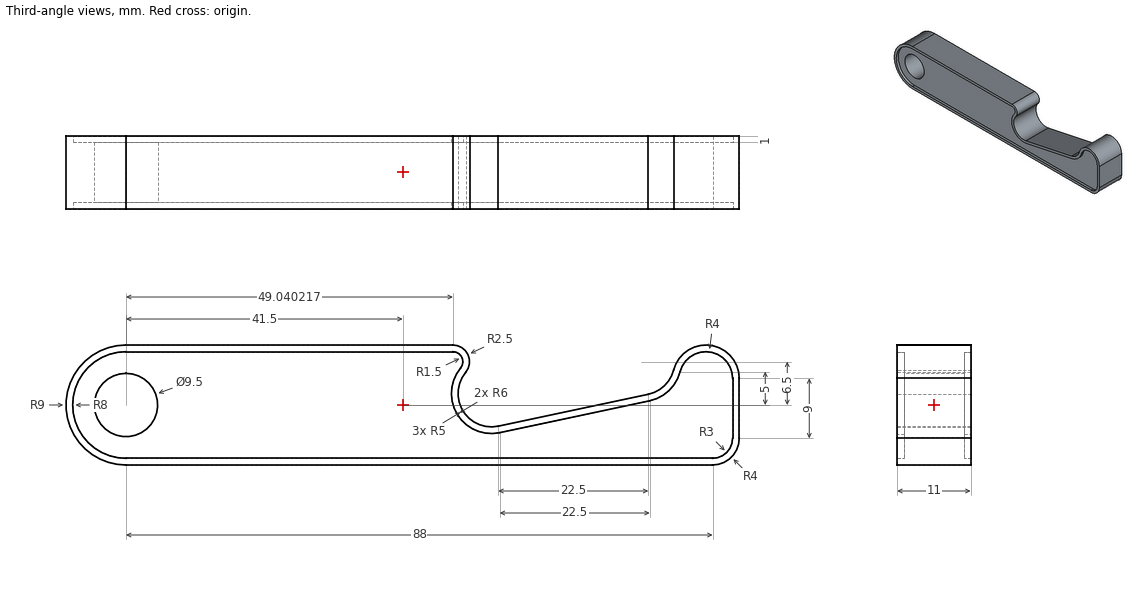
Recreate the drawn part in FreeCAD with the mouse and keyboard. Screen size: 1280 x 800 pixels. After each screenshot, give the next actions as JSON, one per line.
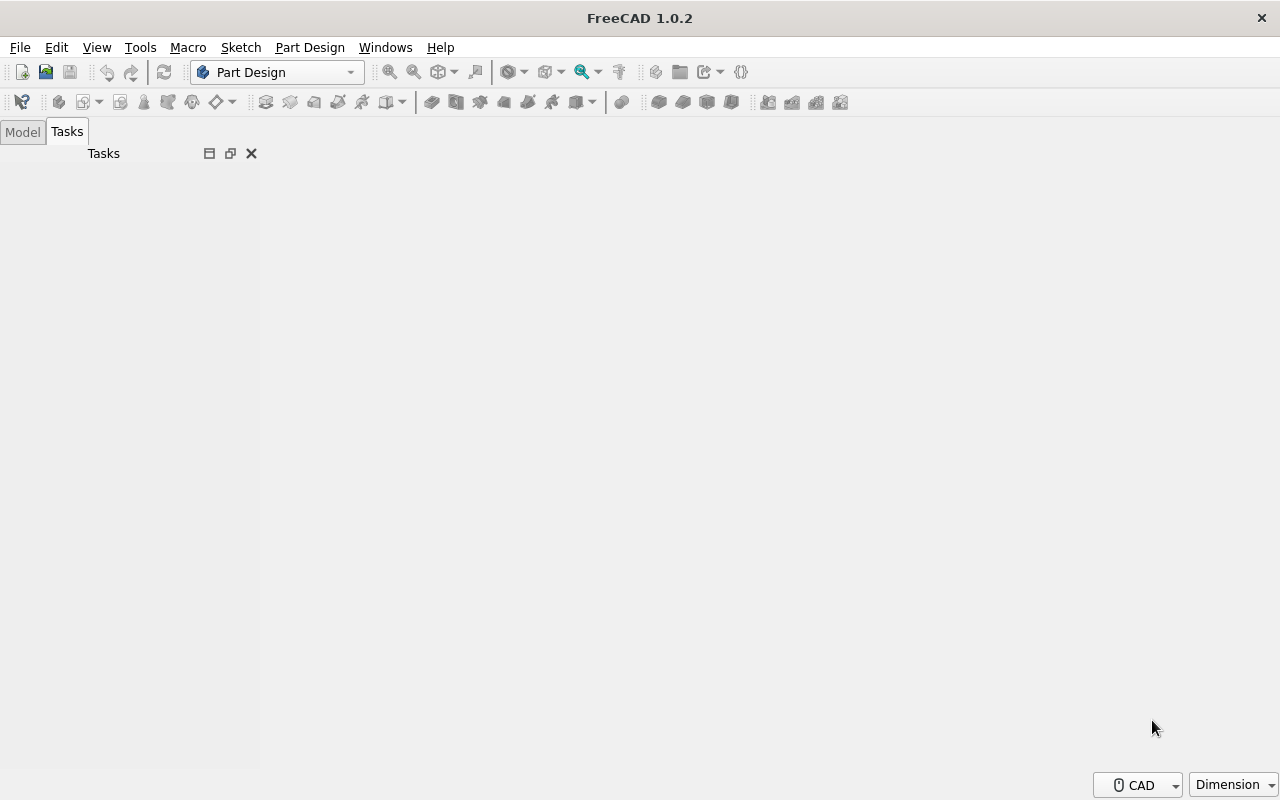
{"action": "left_click", "coordinate": [700, 72]}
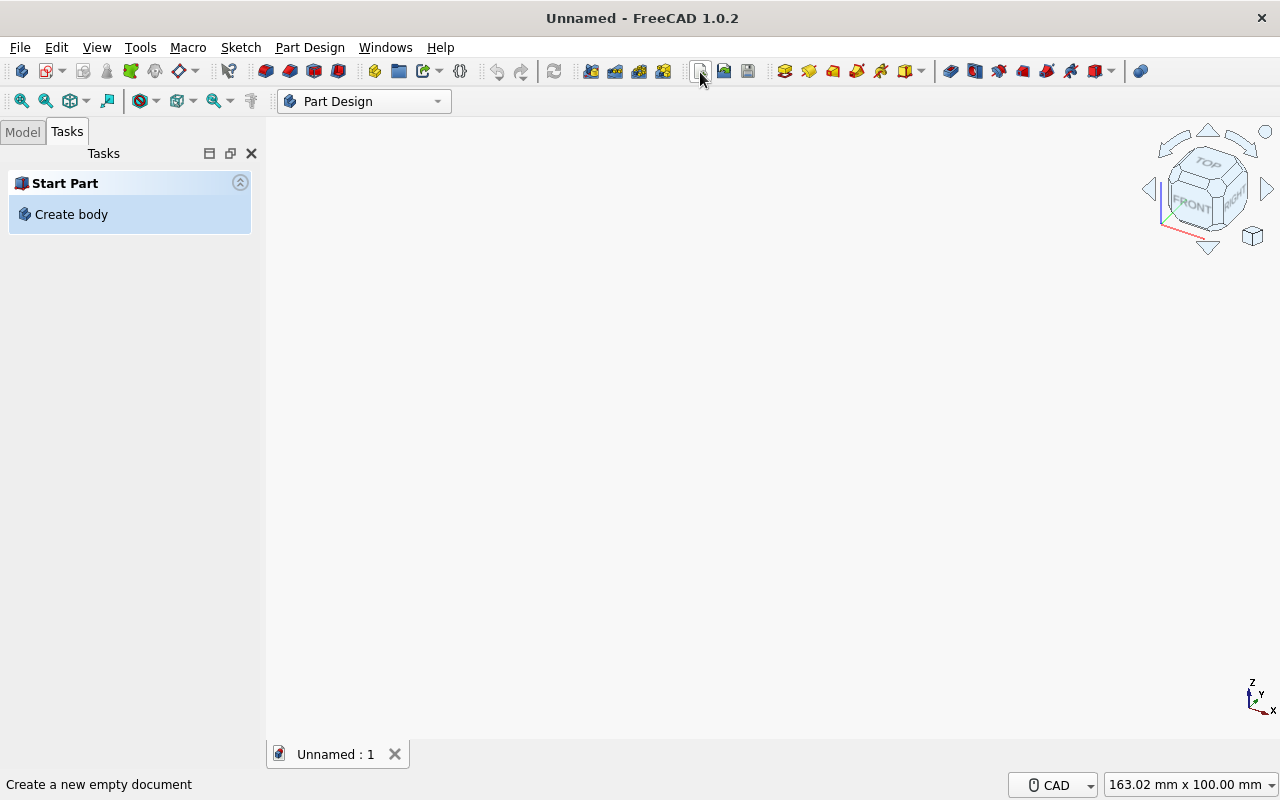
{"action": "left_click", "coordinate": [46, 72]}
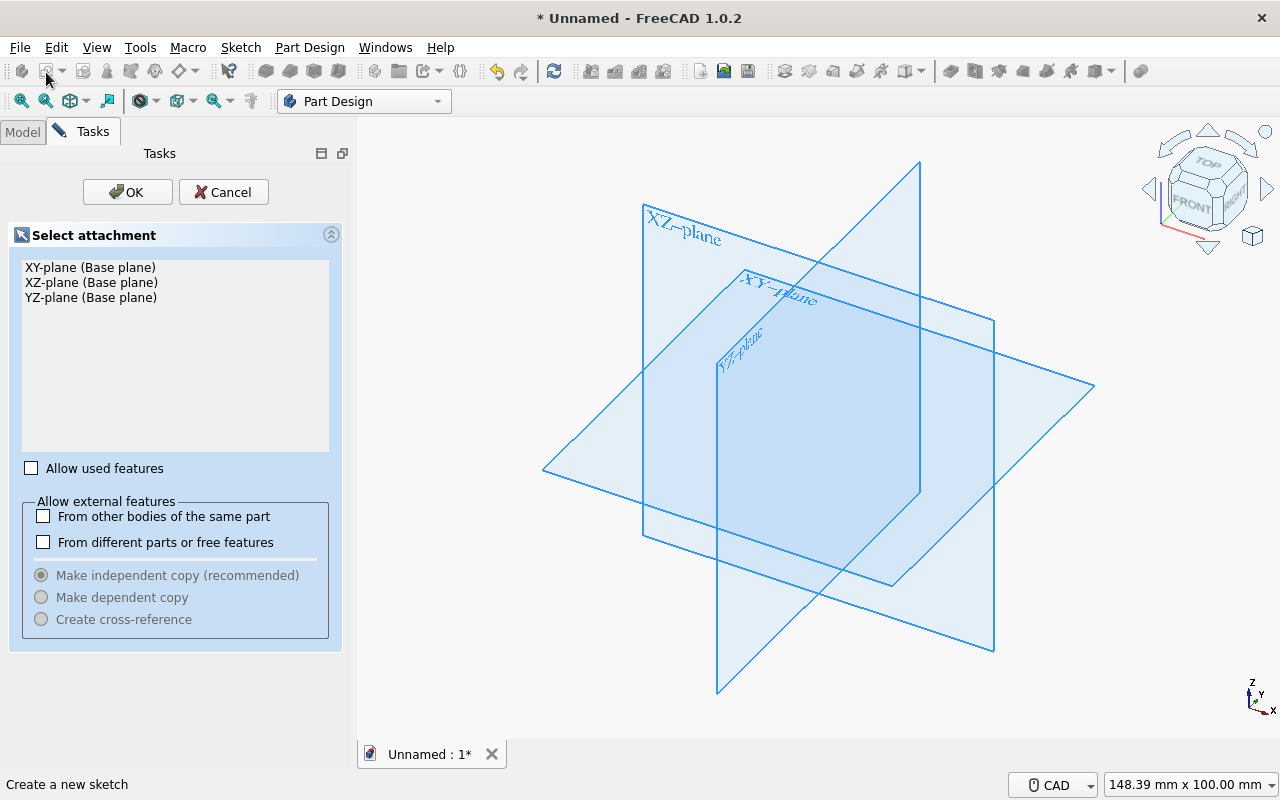
{"action": "left_click", "coordinate": [82, 282]}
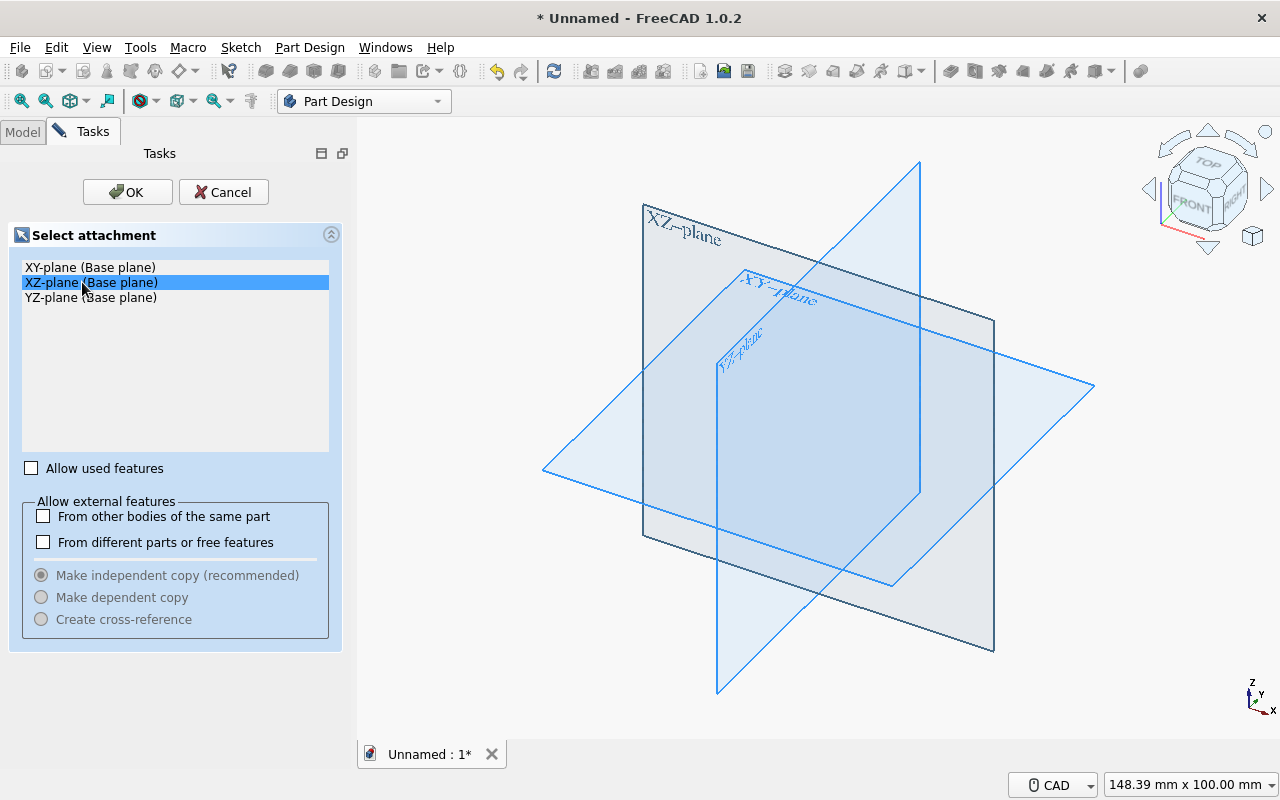
{"action": "left_click", "coordinate": [128, 192]}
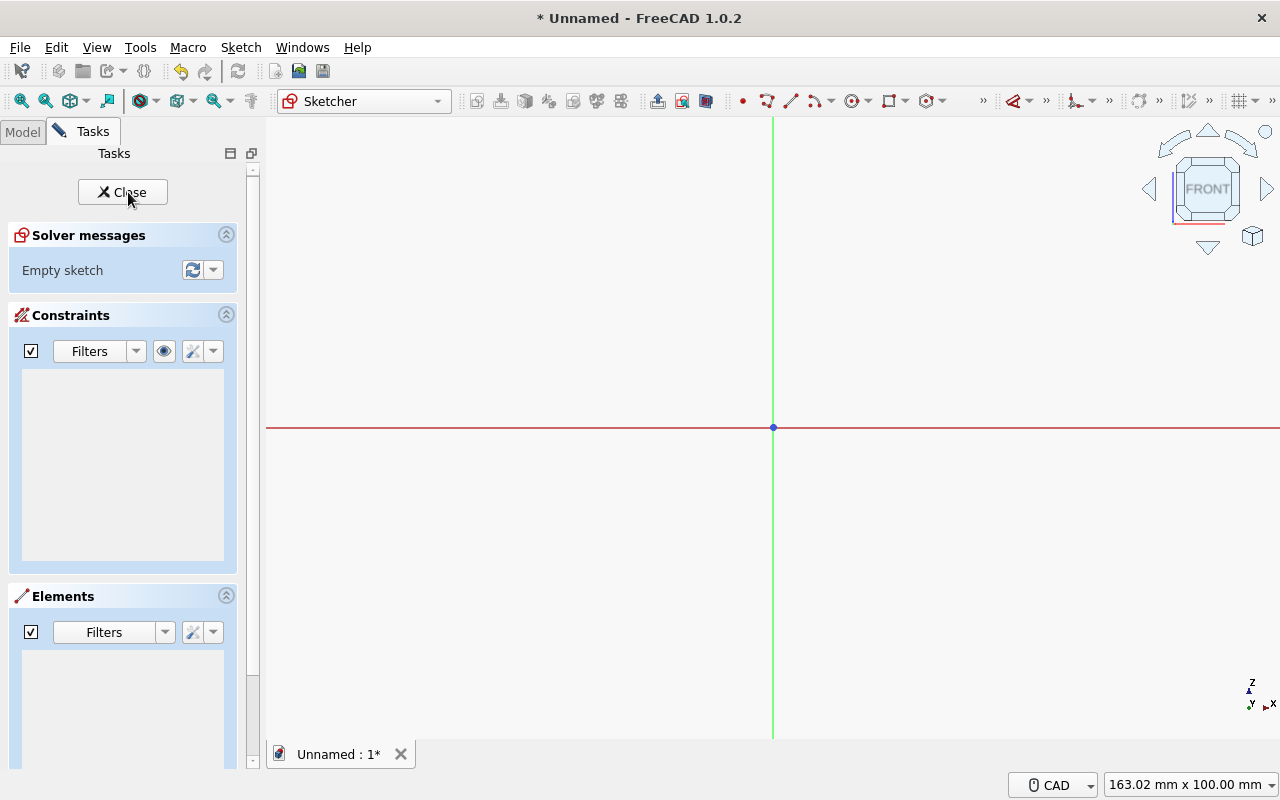
{"action": "left_click", "coordinate": [792, 102]}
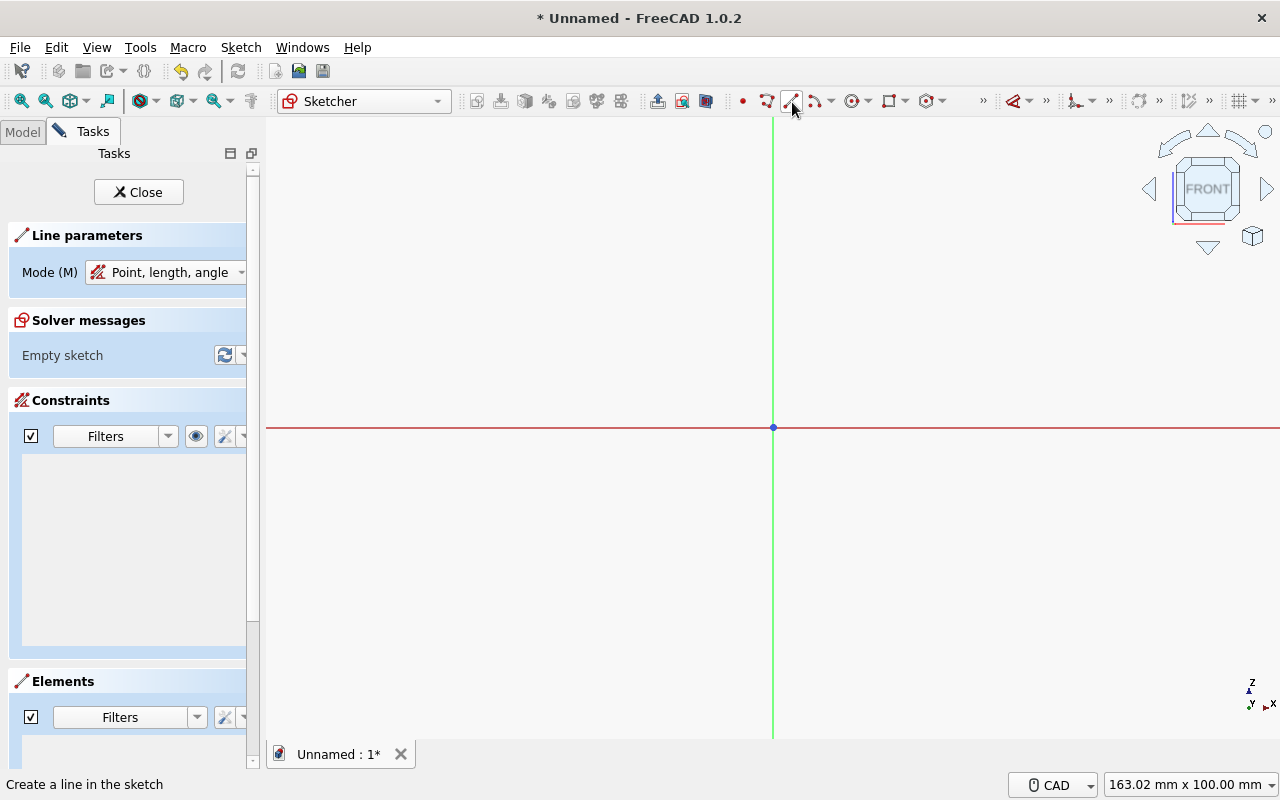
{"action": "left_click", "coordinate": [1062, 484]}
{"action": "left_click", "coordinate": [515, 484]}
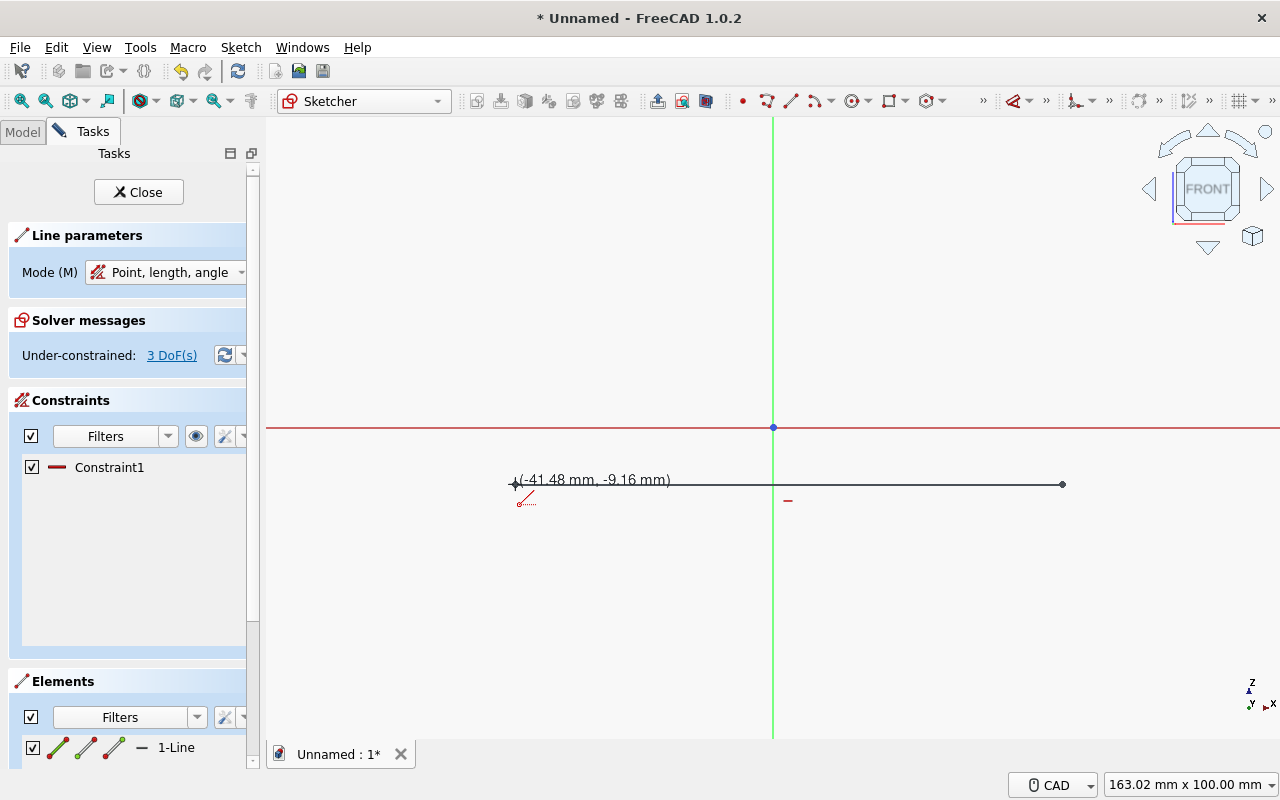
{"action": "left_click", "coordinate": [515, 372]}
{"action": "left_click", "coordinate": [820, 372]}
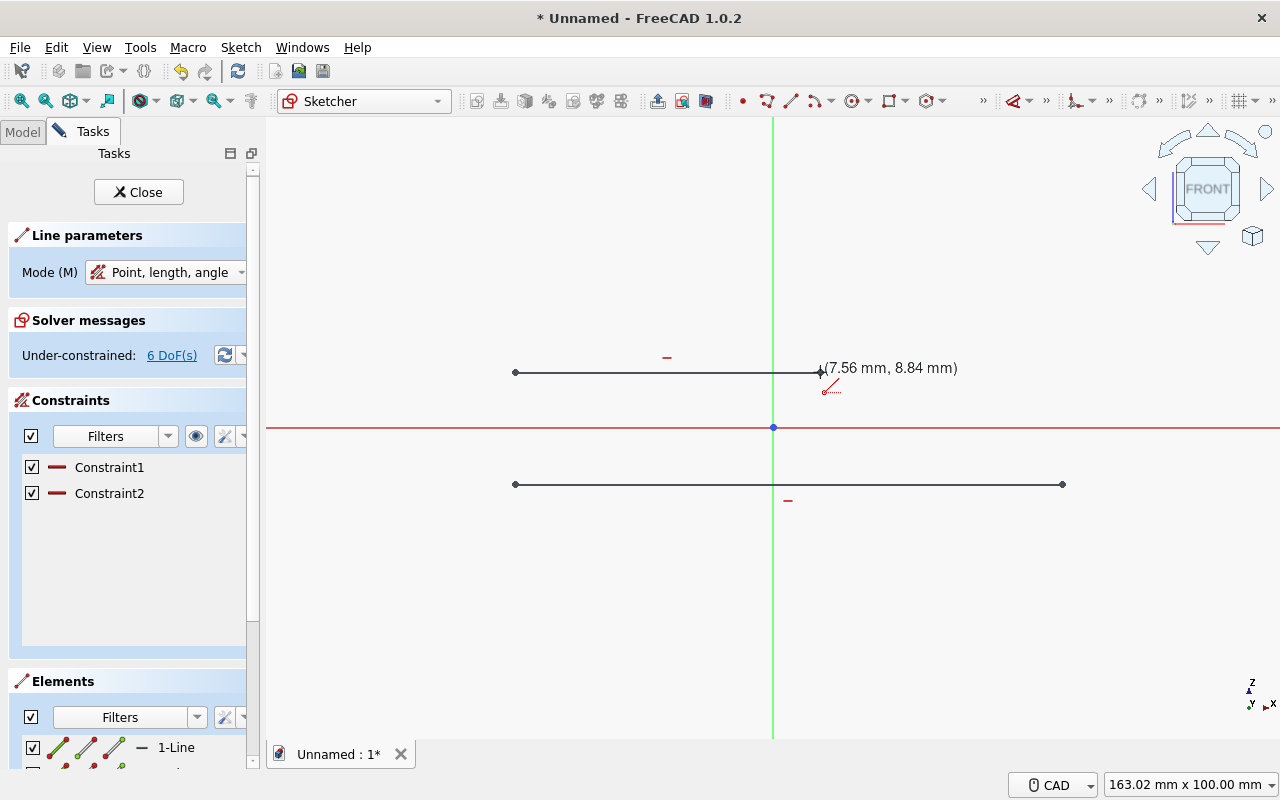
{"action": "left_click", "coordinate": [862, 448]}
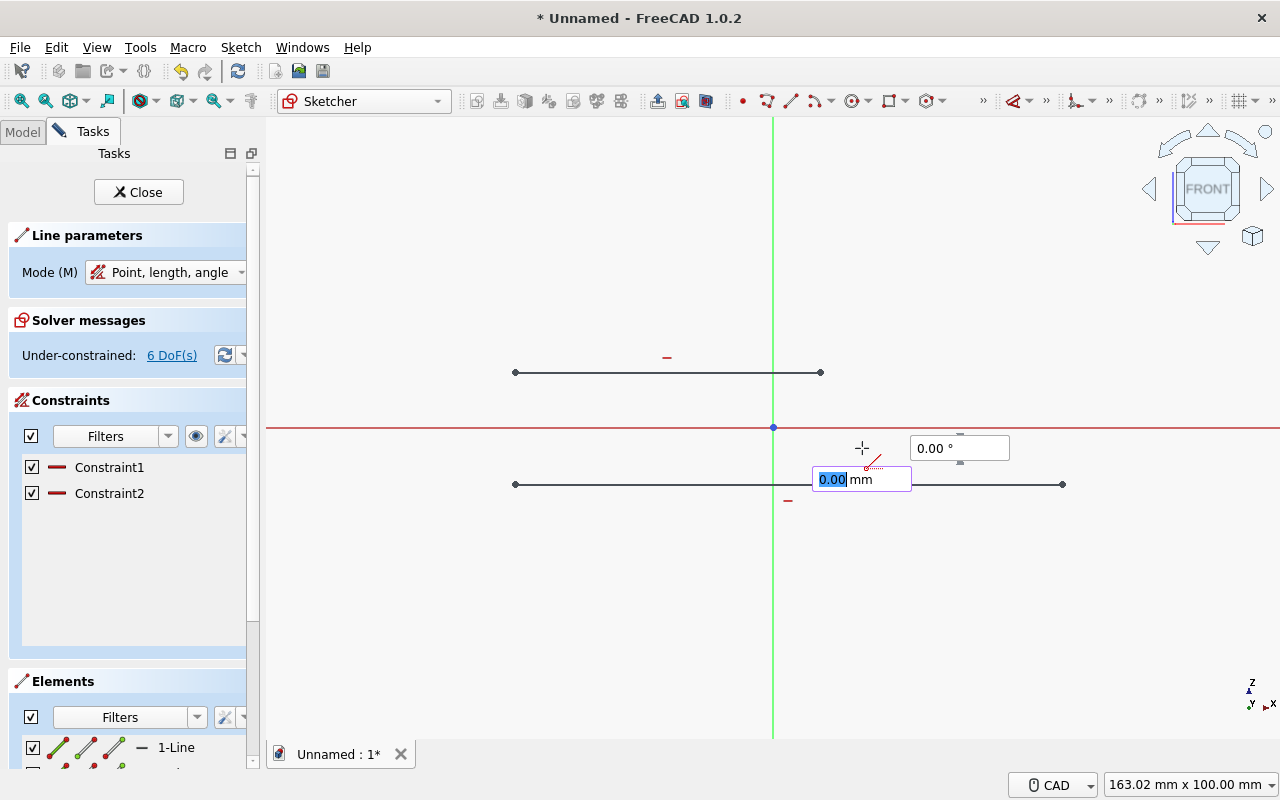
{"action": "scroll", "coordinate": [1002, 418], "scroll_direction": "up", "scroll_amount": 3}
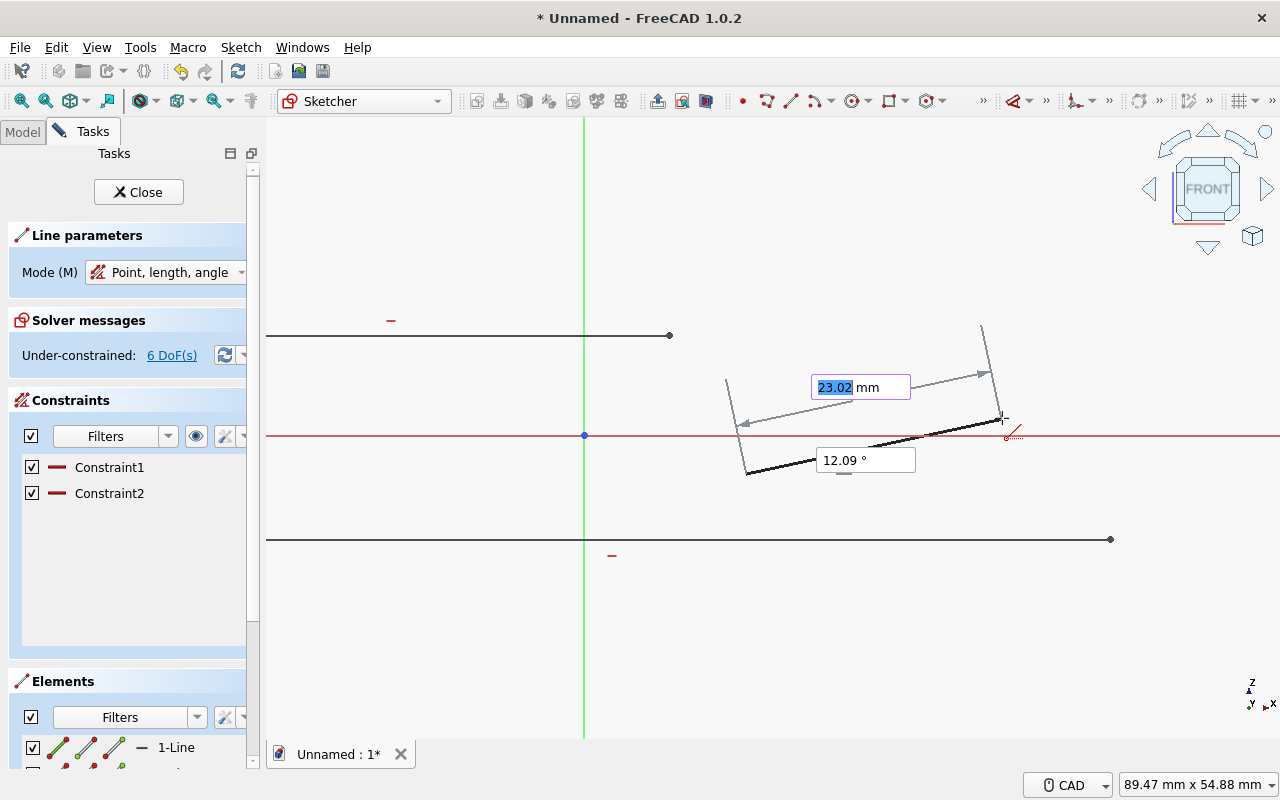
{"action": "left_click", "coordinate": [1002, 418]}